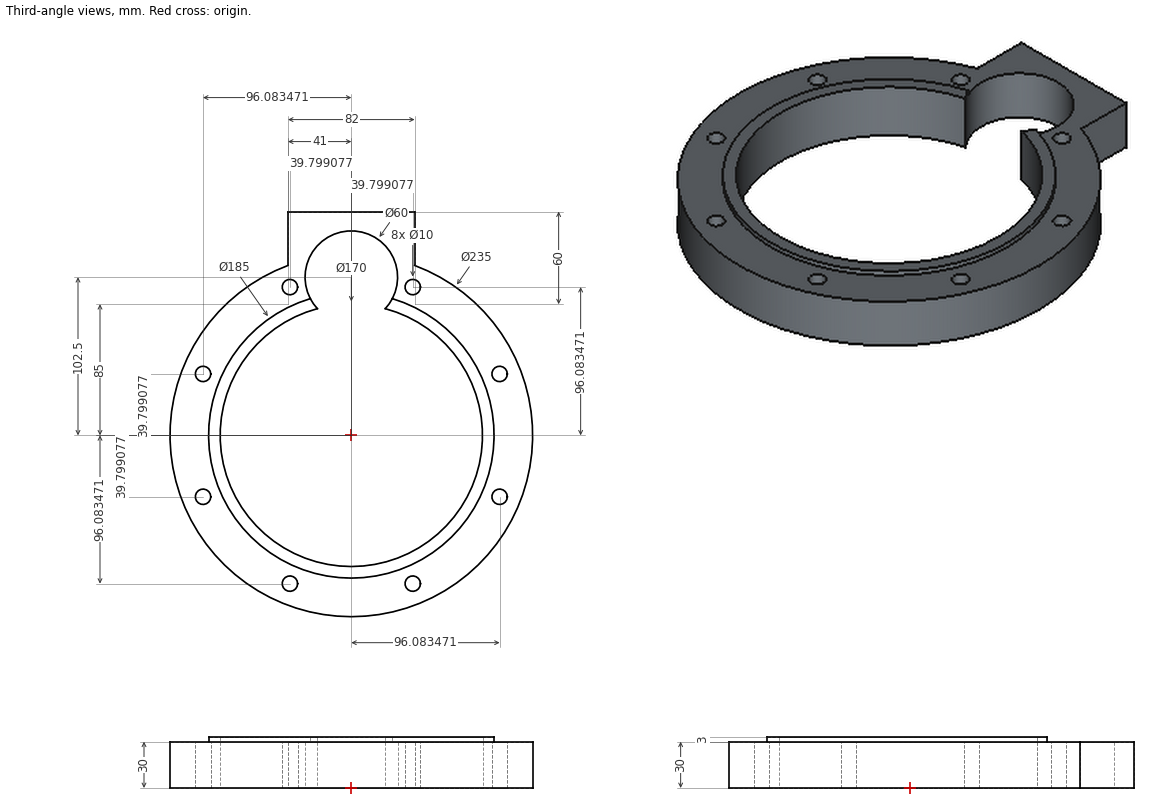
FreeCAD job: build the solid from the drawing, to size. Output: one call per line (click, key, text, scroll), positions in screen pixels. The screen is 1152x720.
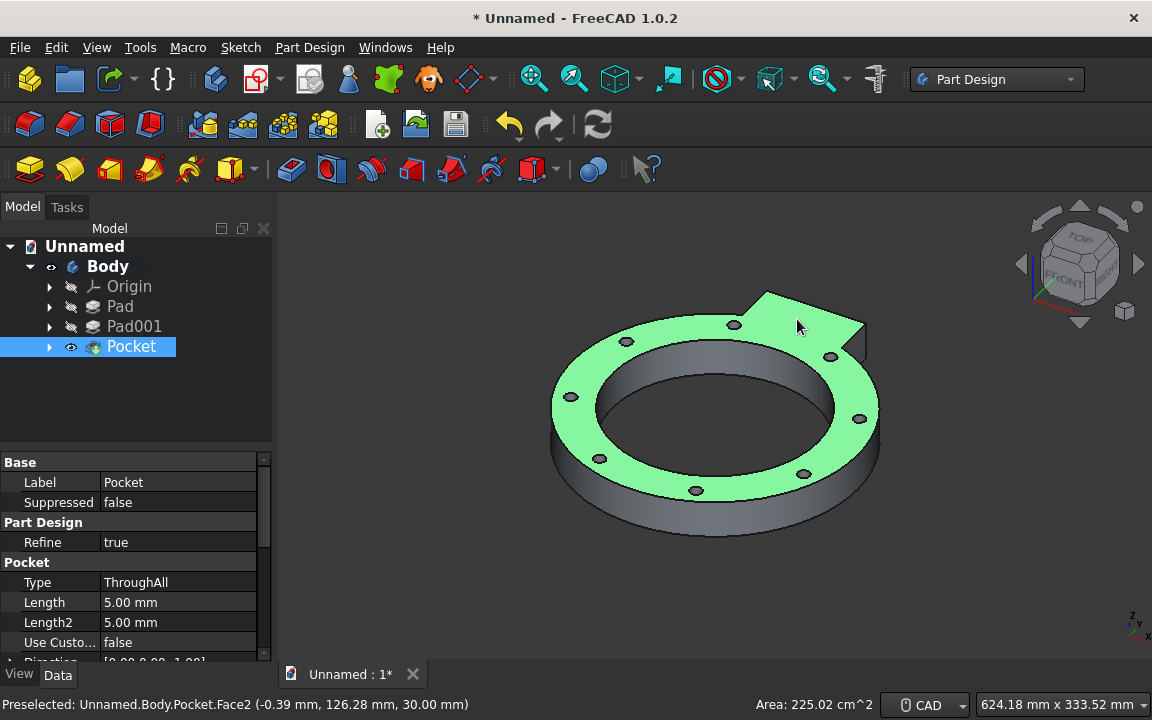
click(256, 80)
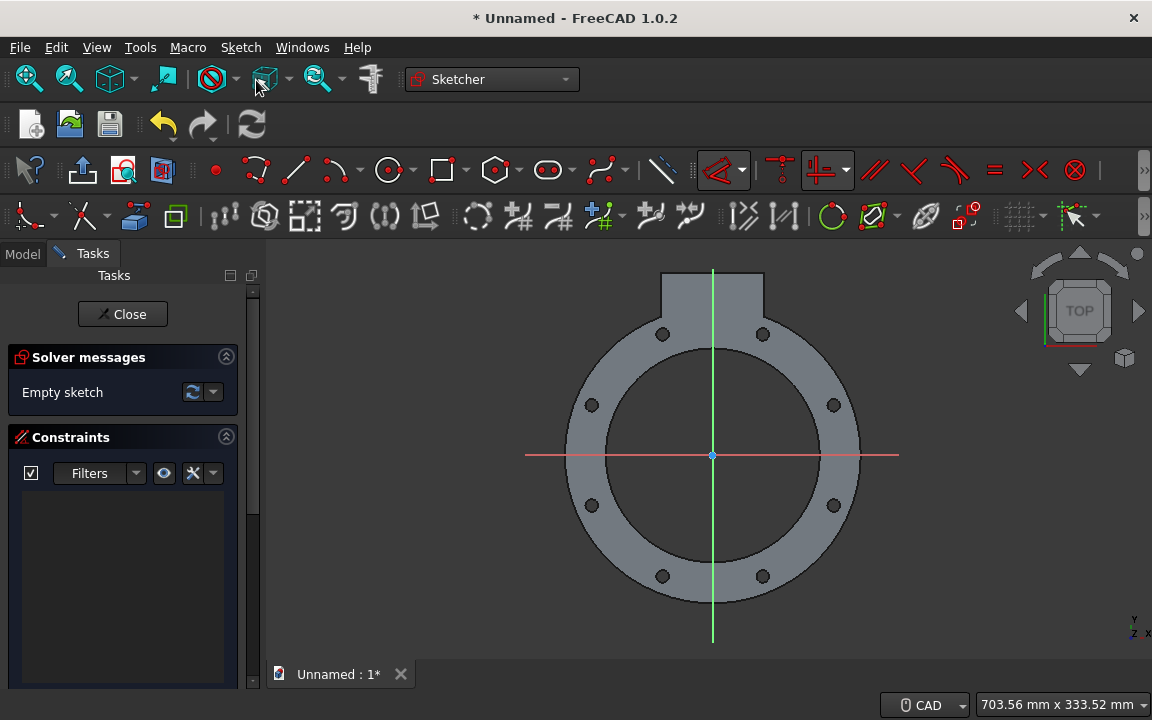
click(390, 170)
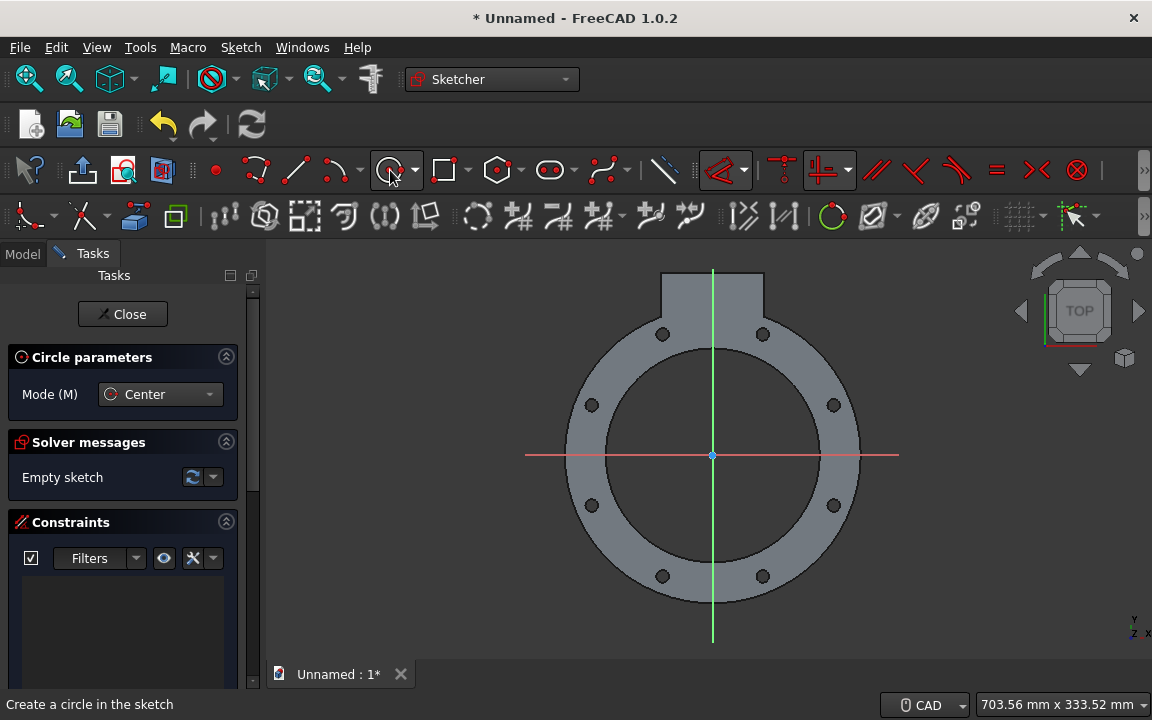
click(713, 455)
move(795, 373)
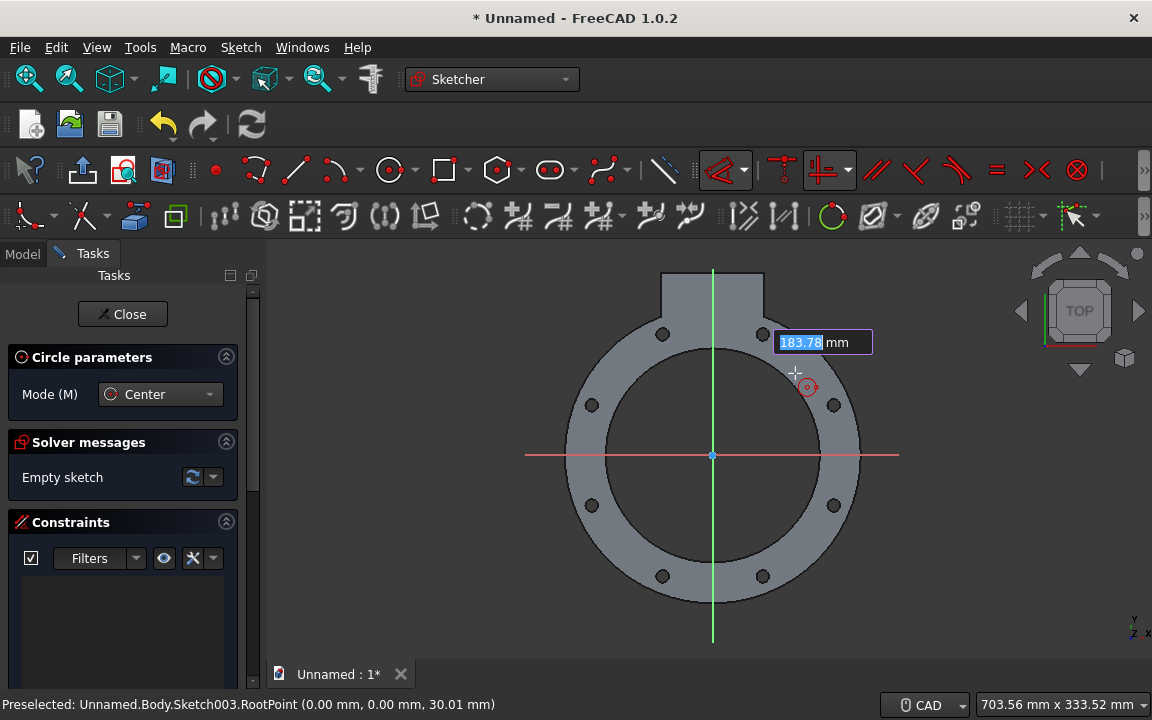
text(185)
key(Return)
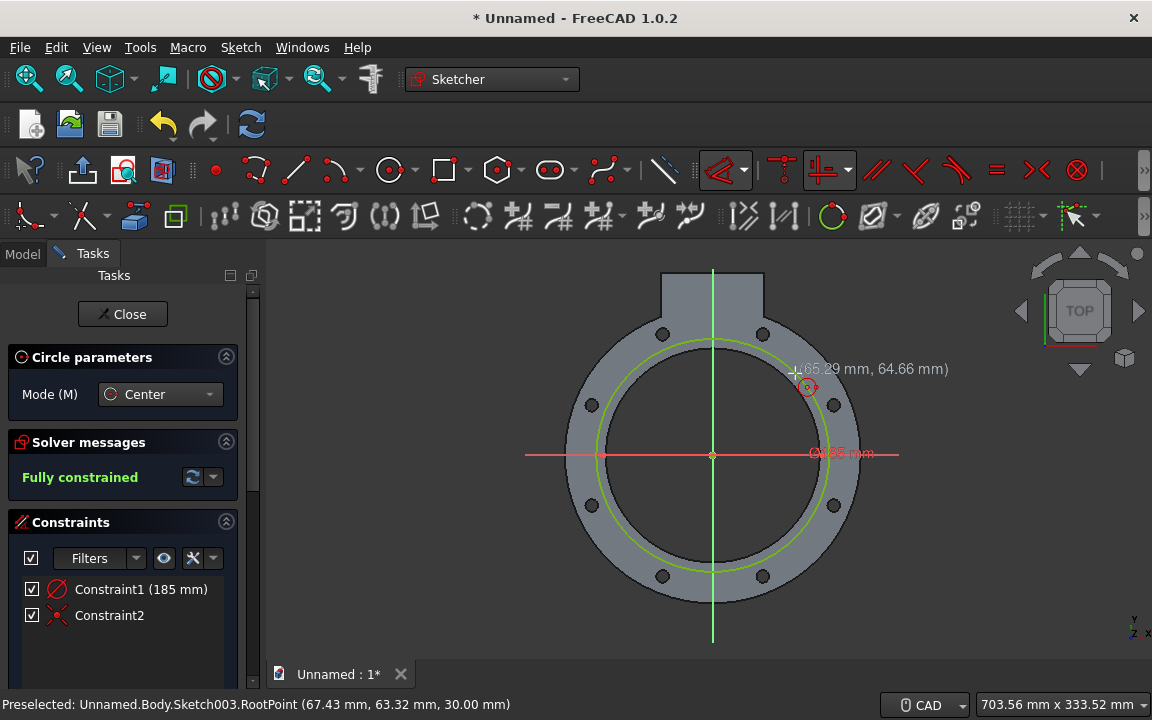
click(713, 455)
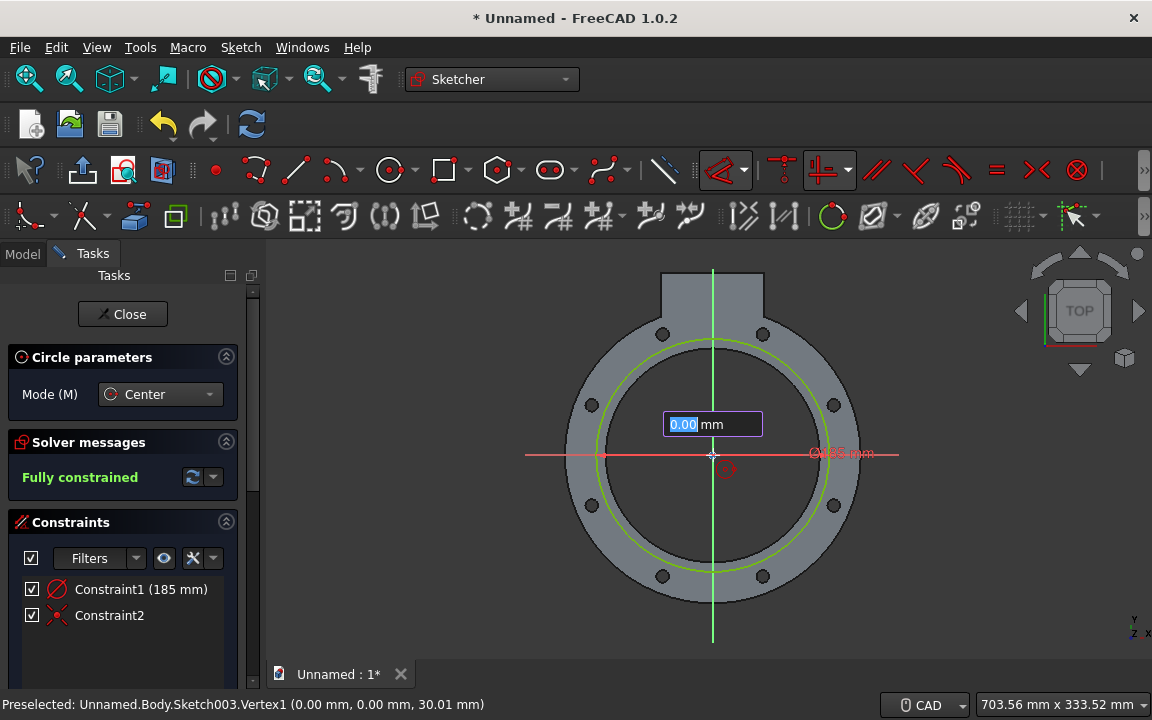
scroll(788, 380, up, 3)
move(788, 379)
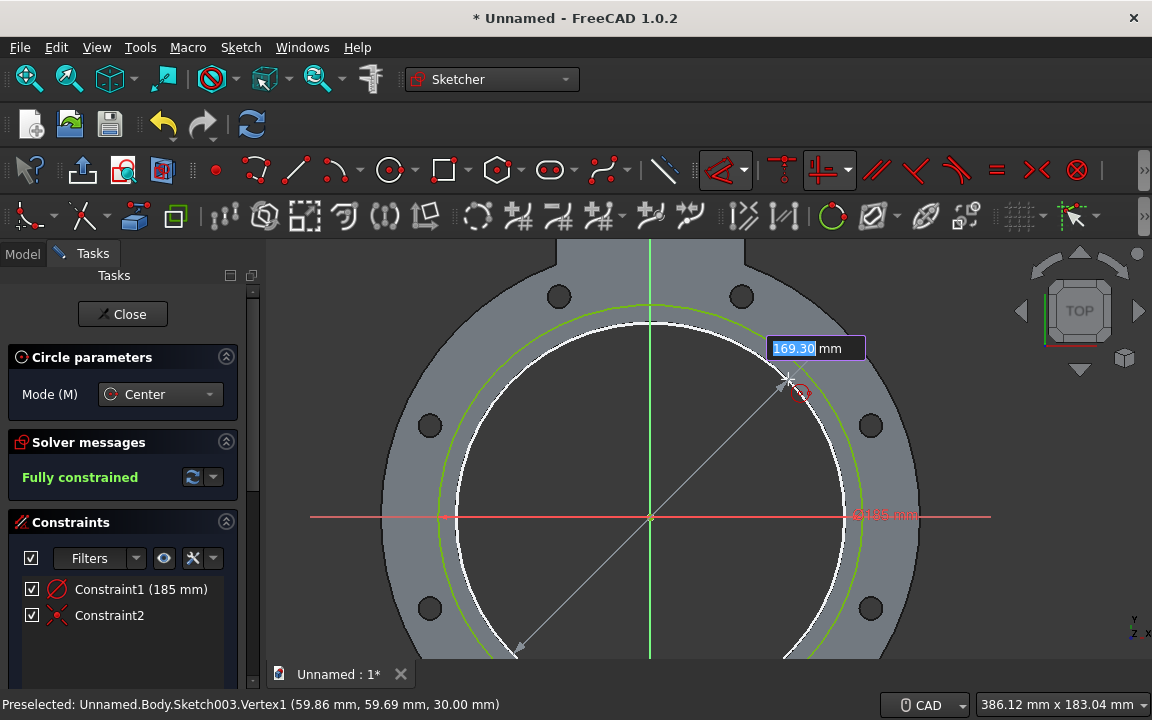
text(170)
key(Return)
key(Escape)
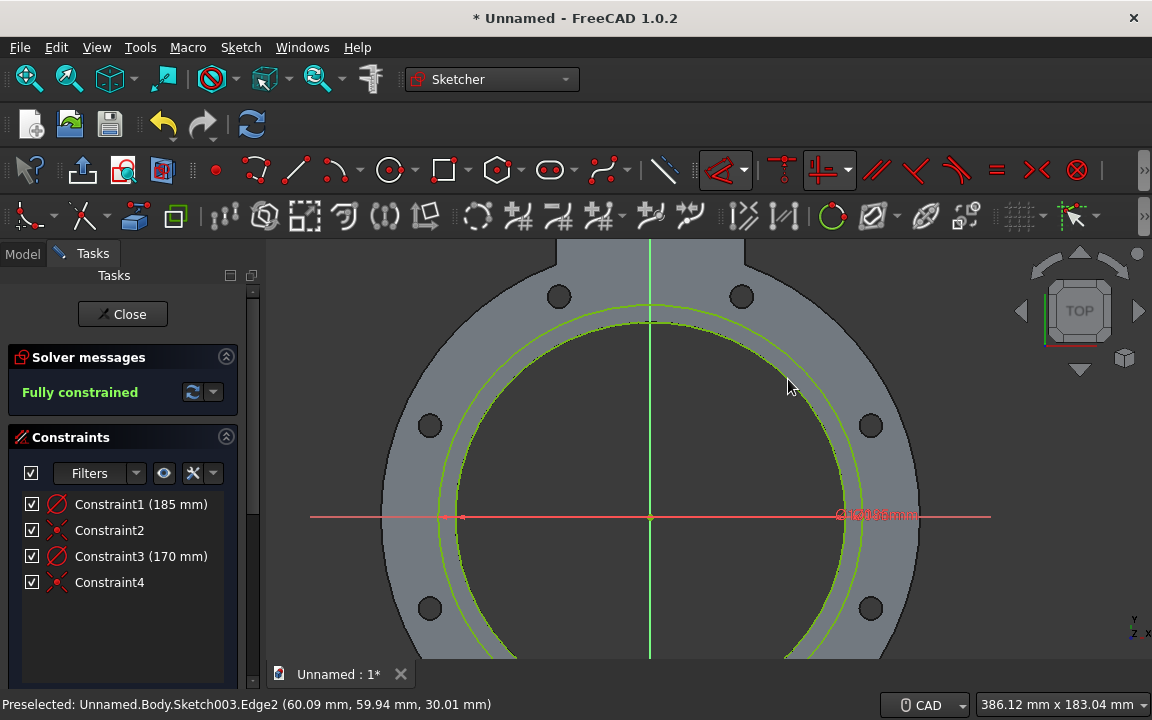
click(123, 314)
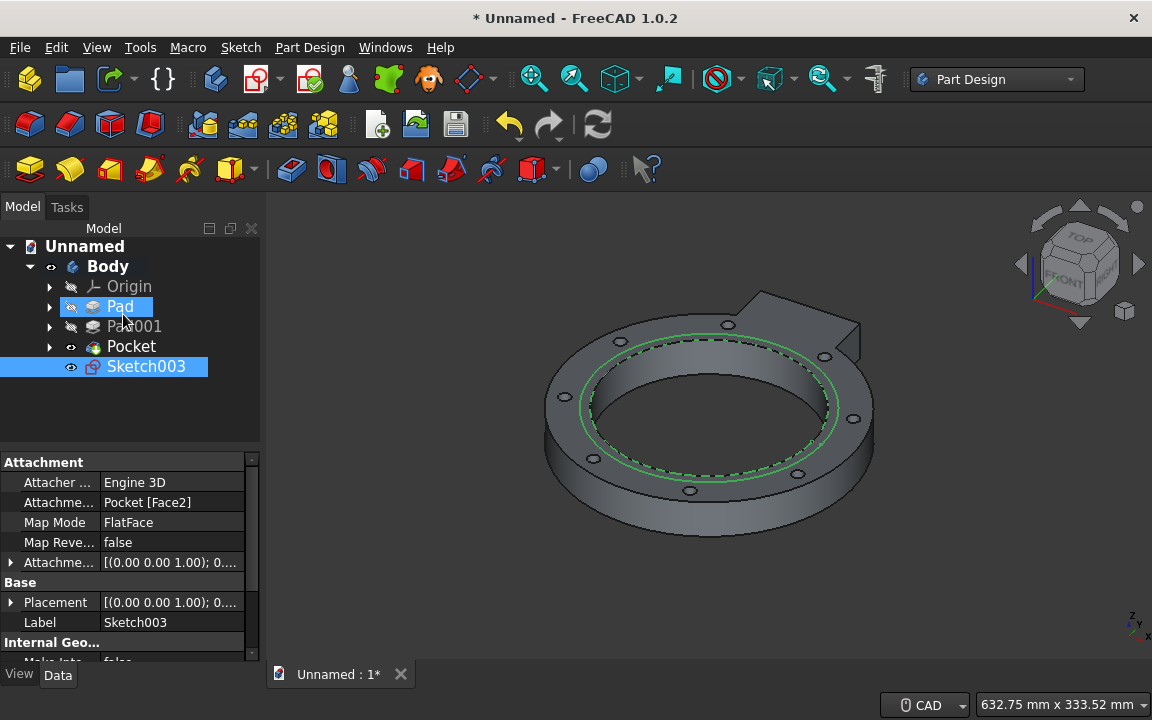
click(30, 170)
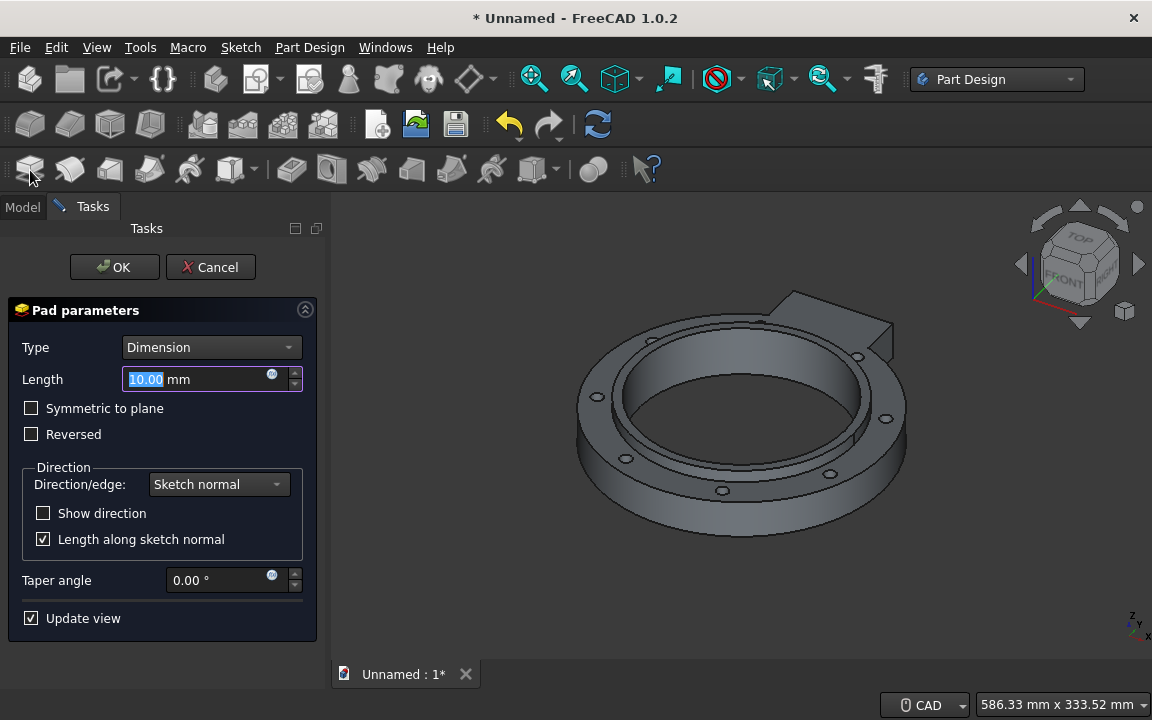
text(3)
key(Tab)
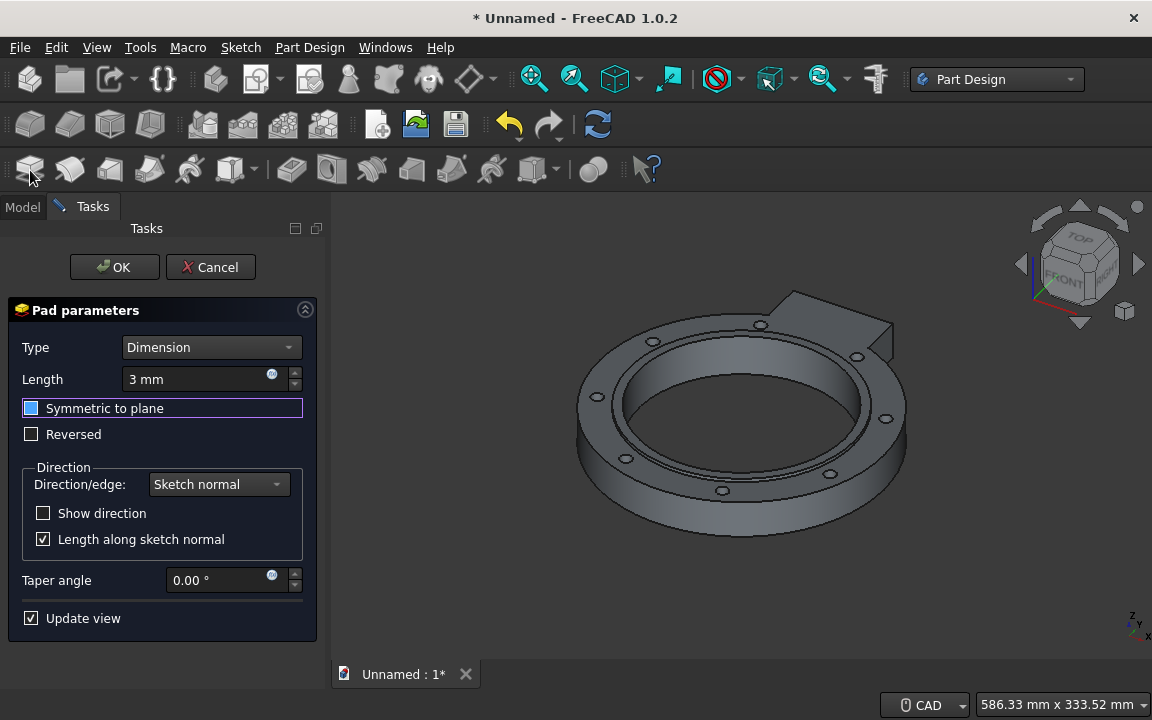
click(115, 267)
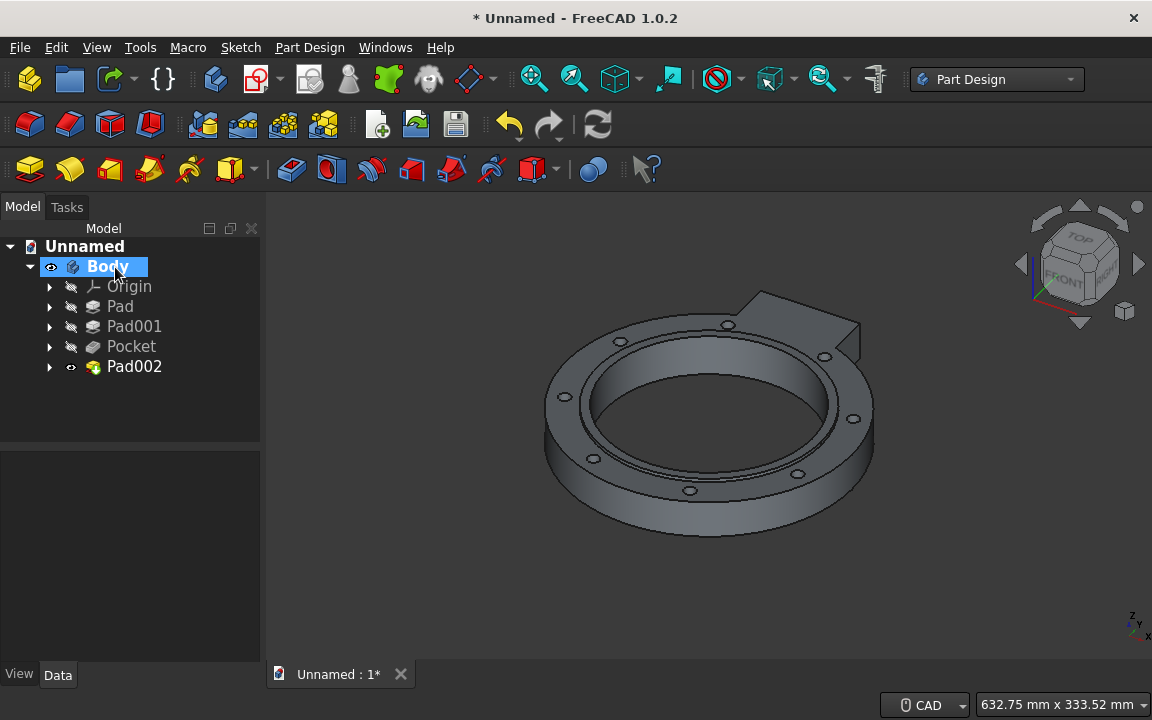
click(256, 80)